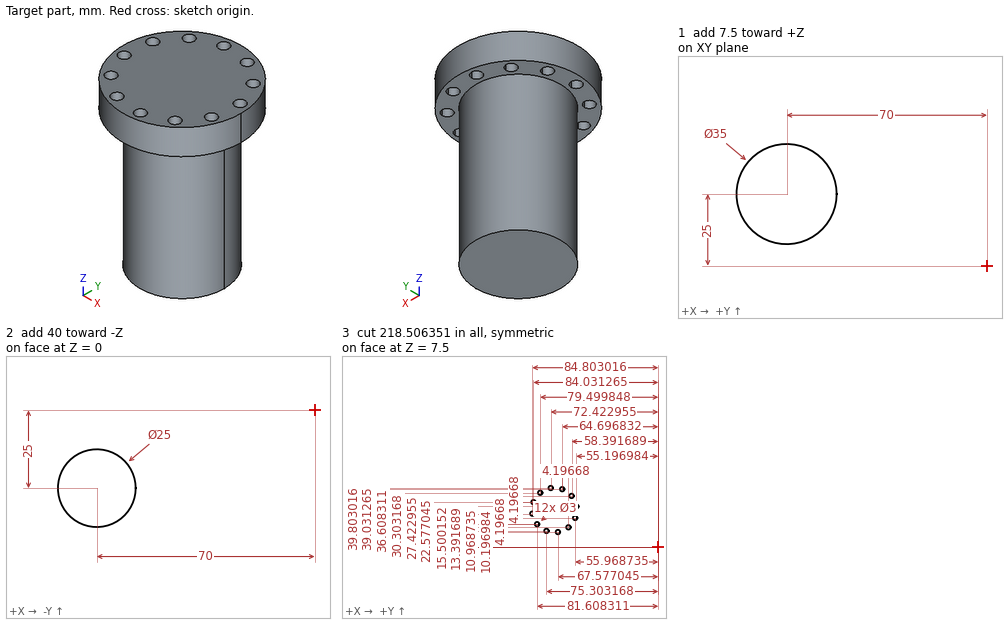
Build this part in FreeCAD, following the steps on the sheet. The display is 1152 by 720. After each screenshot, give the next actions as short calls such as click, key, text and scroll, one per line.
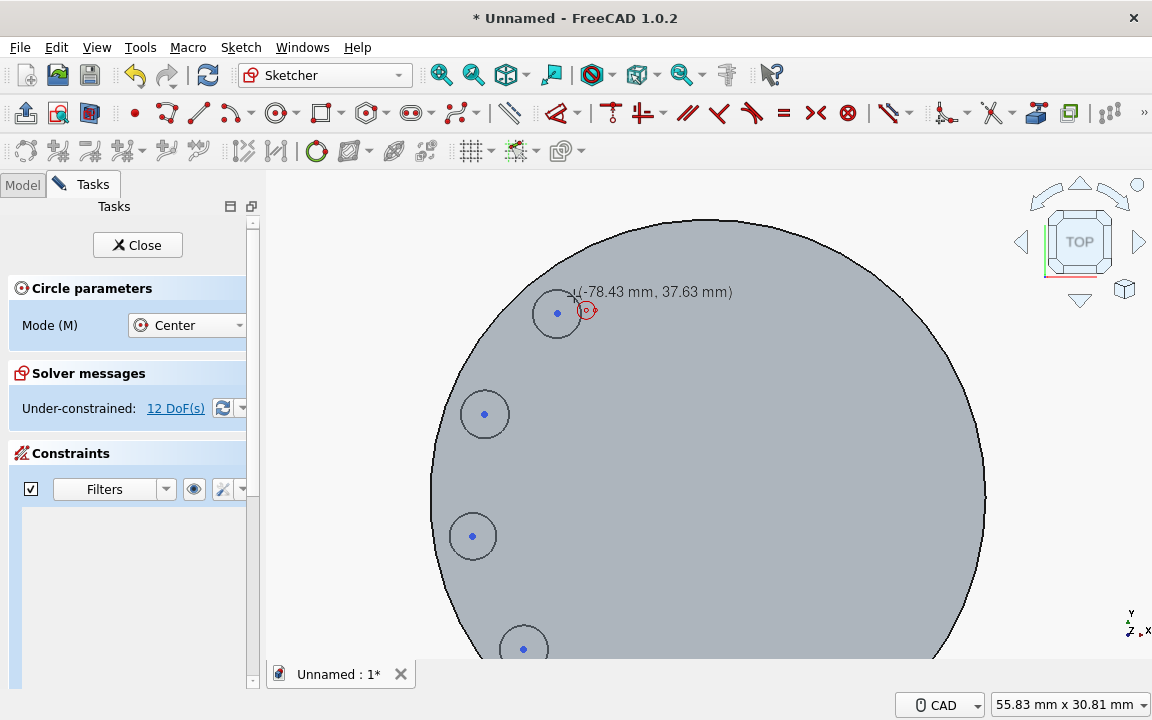
click(669, 262)
click(686, 246)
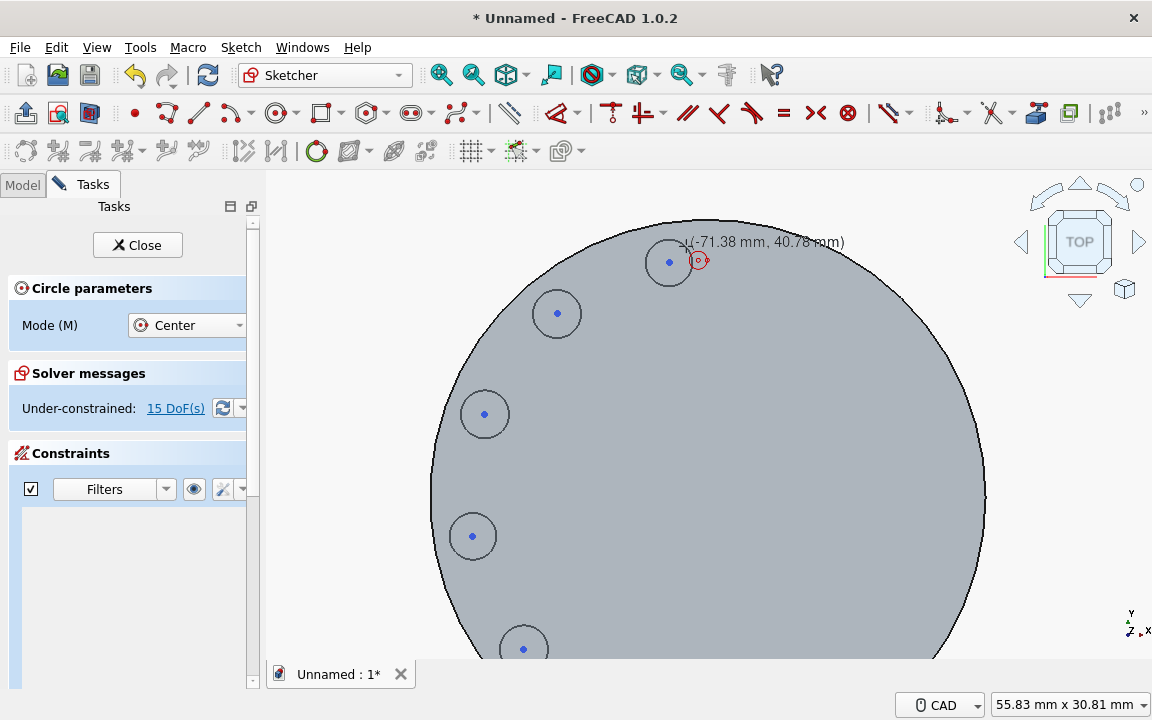
click(792, 275)
click(809, 258)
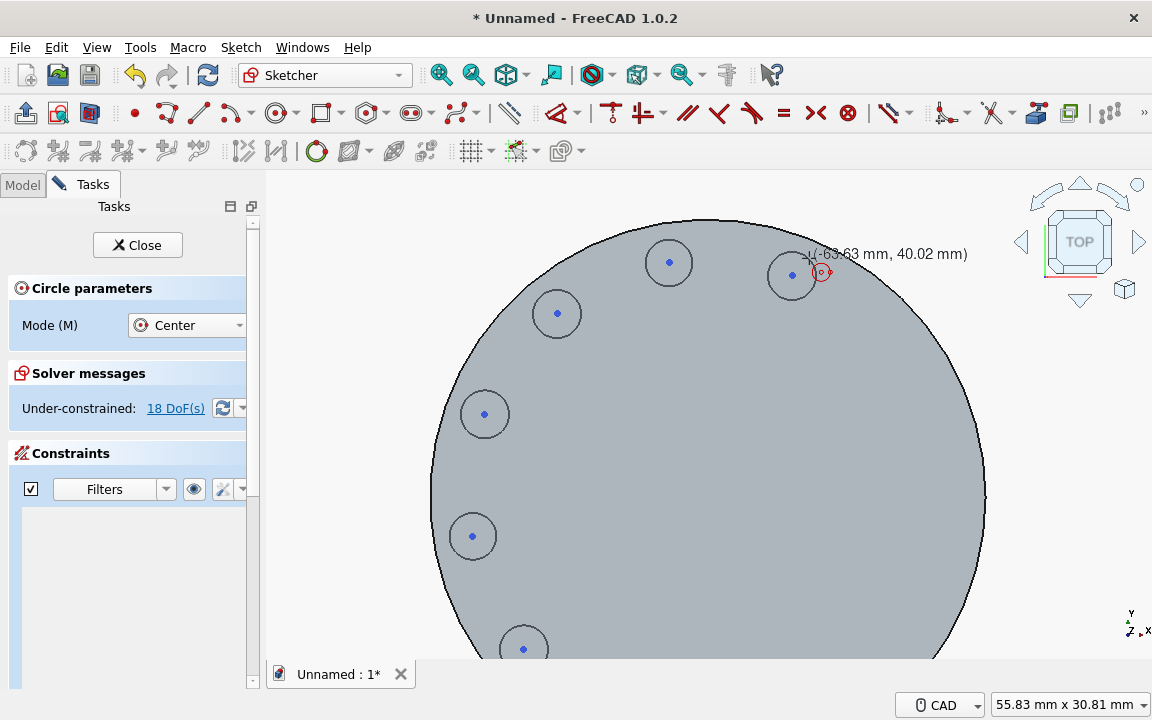
click(892, 347)
click(909, 330)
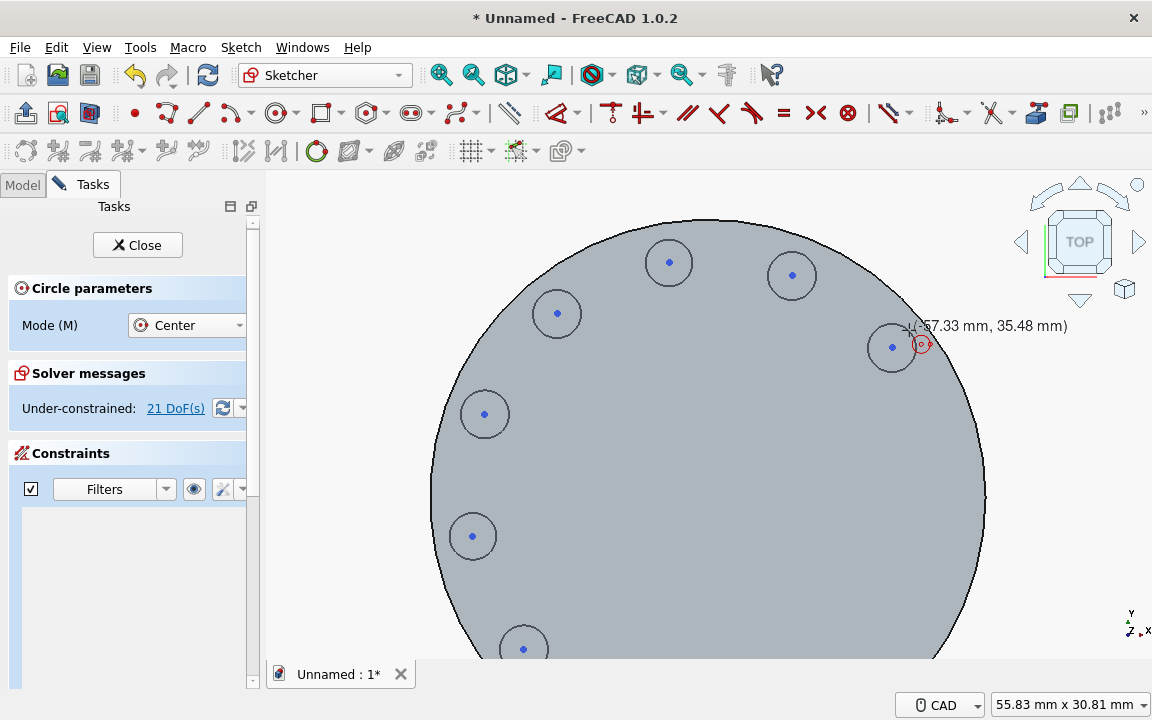
click(943, 459)
click(960, 442)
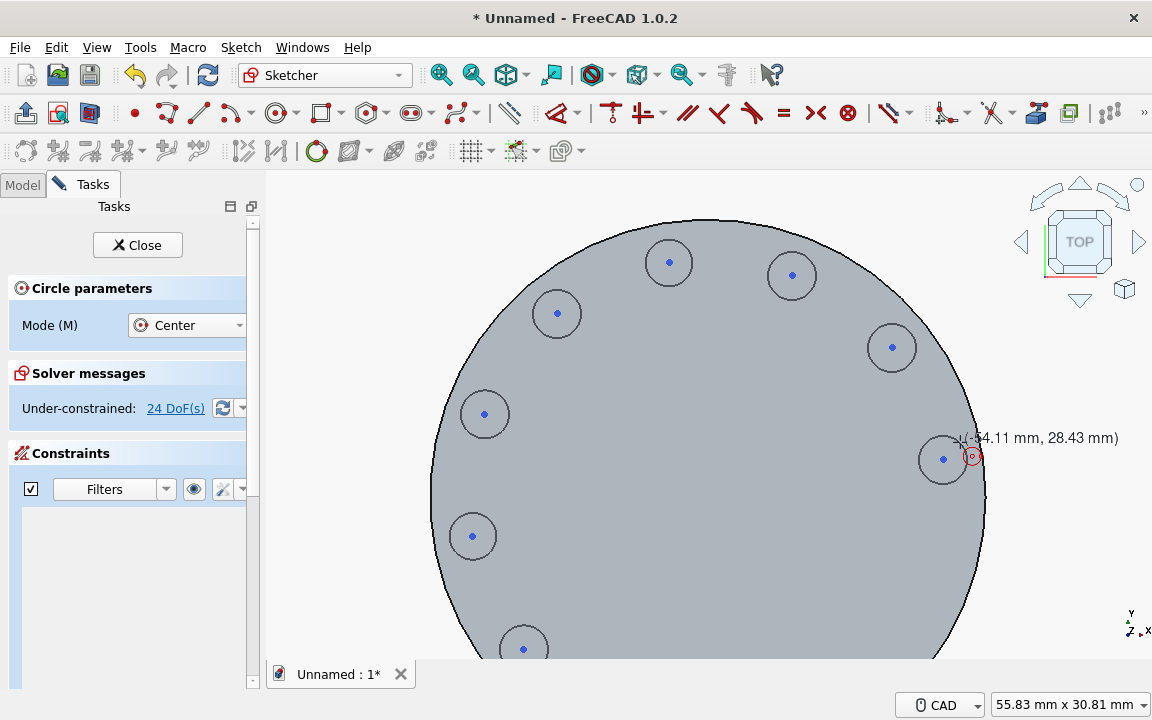
click(931, 582)
click(947, 565)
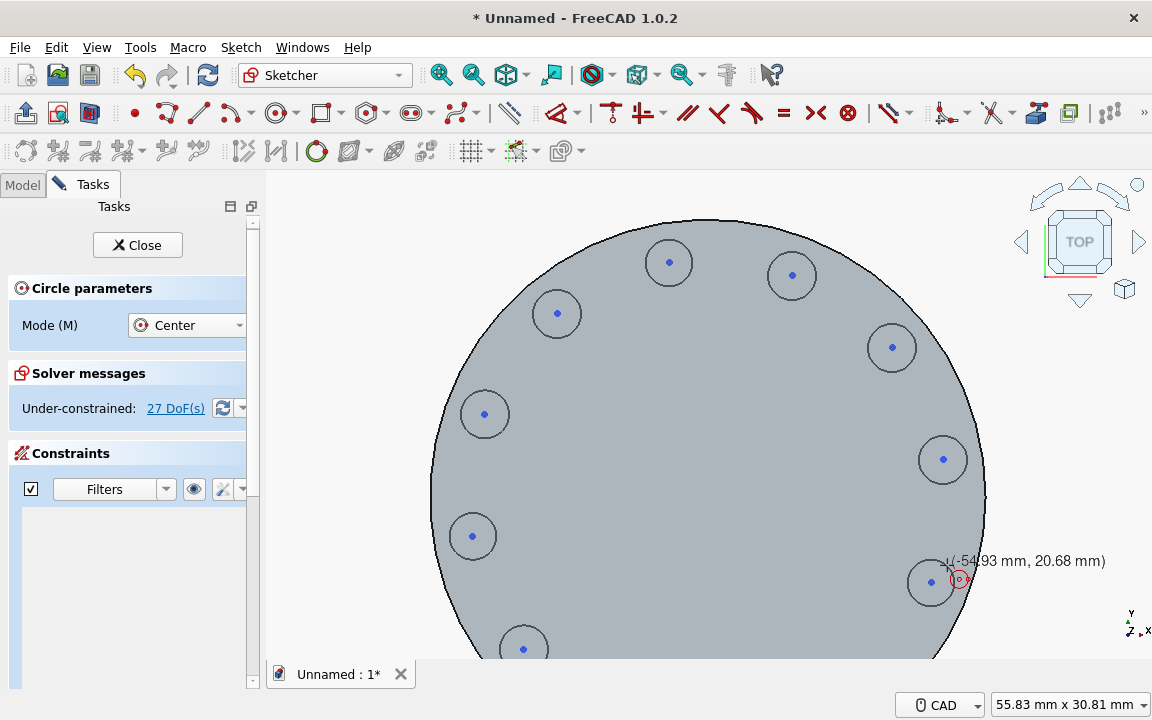
scroll(559, 314, down, 3)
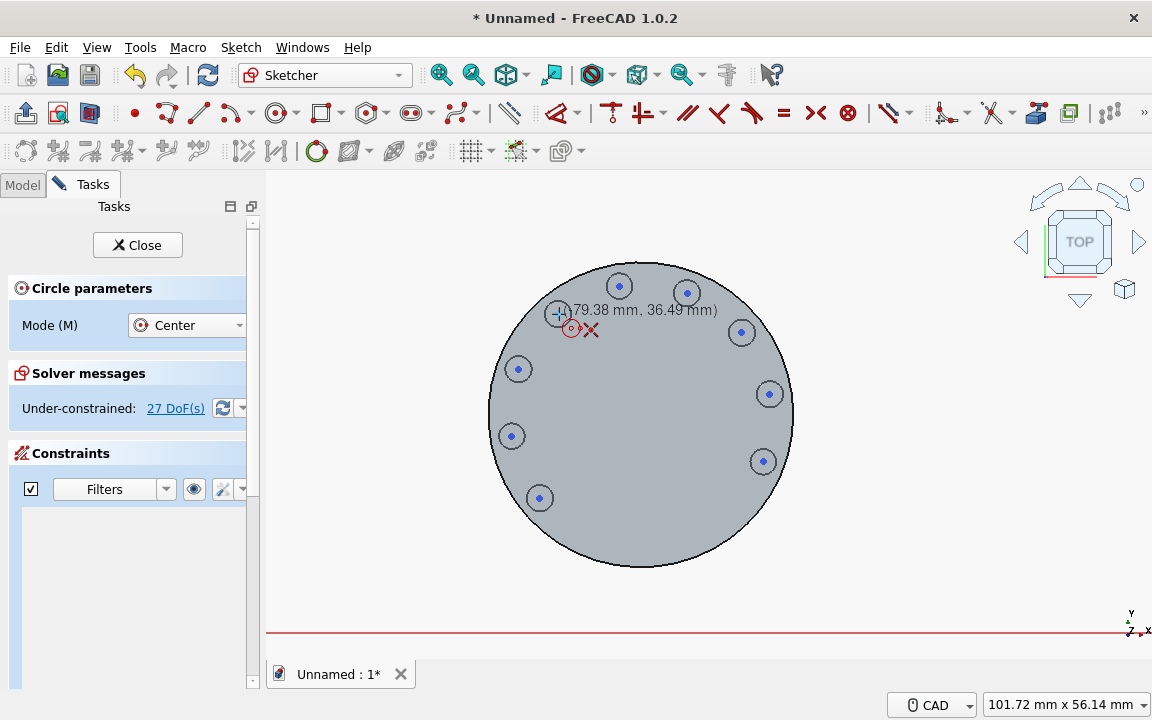
scroll(724, 516, up, 3)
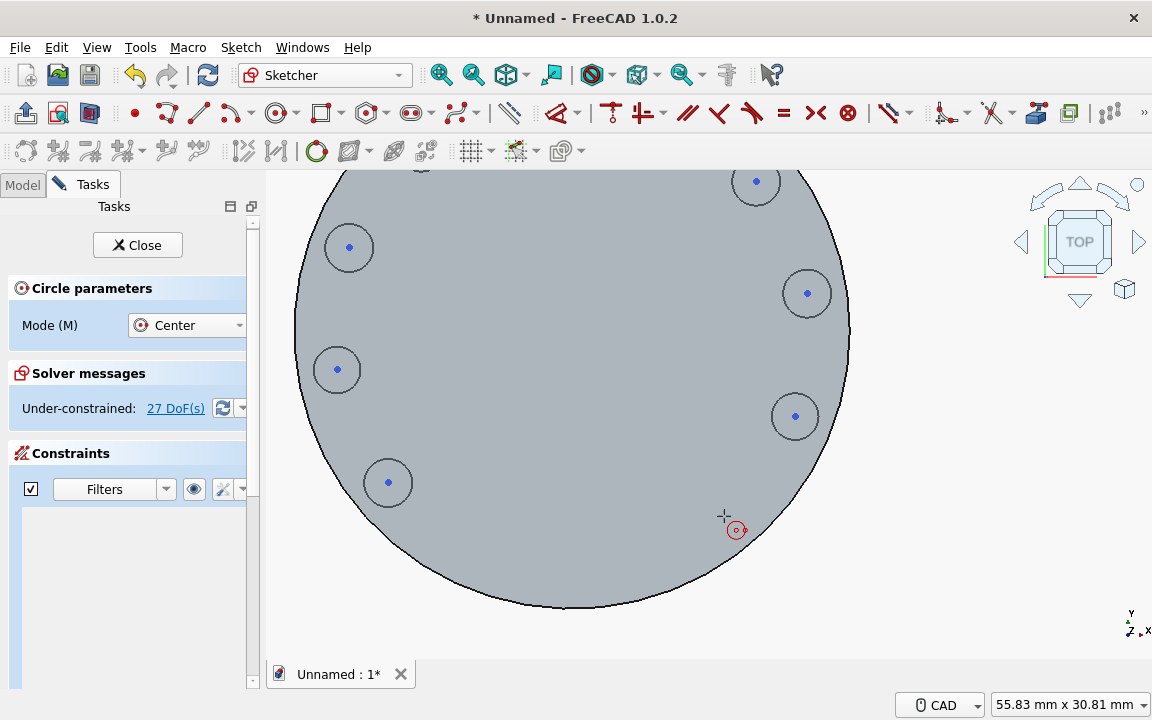
click(723, 515)
click(740, 498)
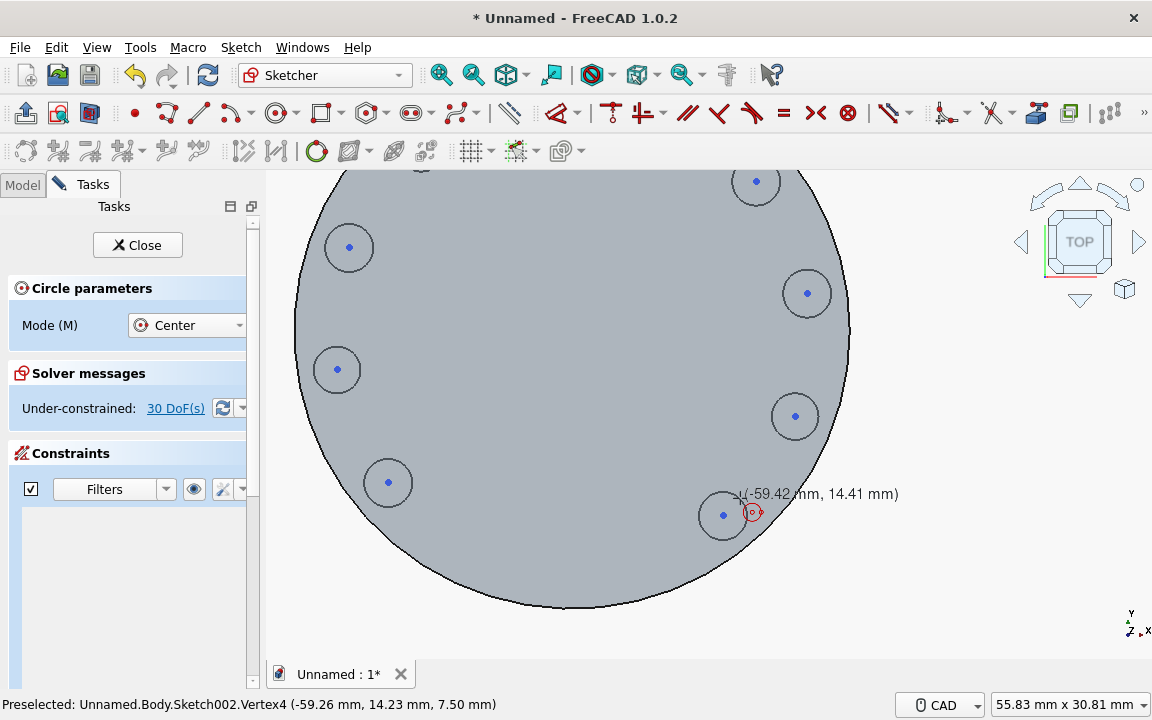
click(611, 566)
click(627, 549)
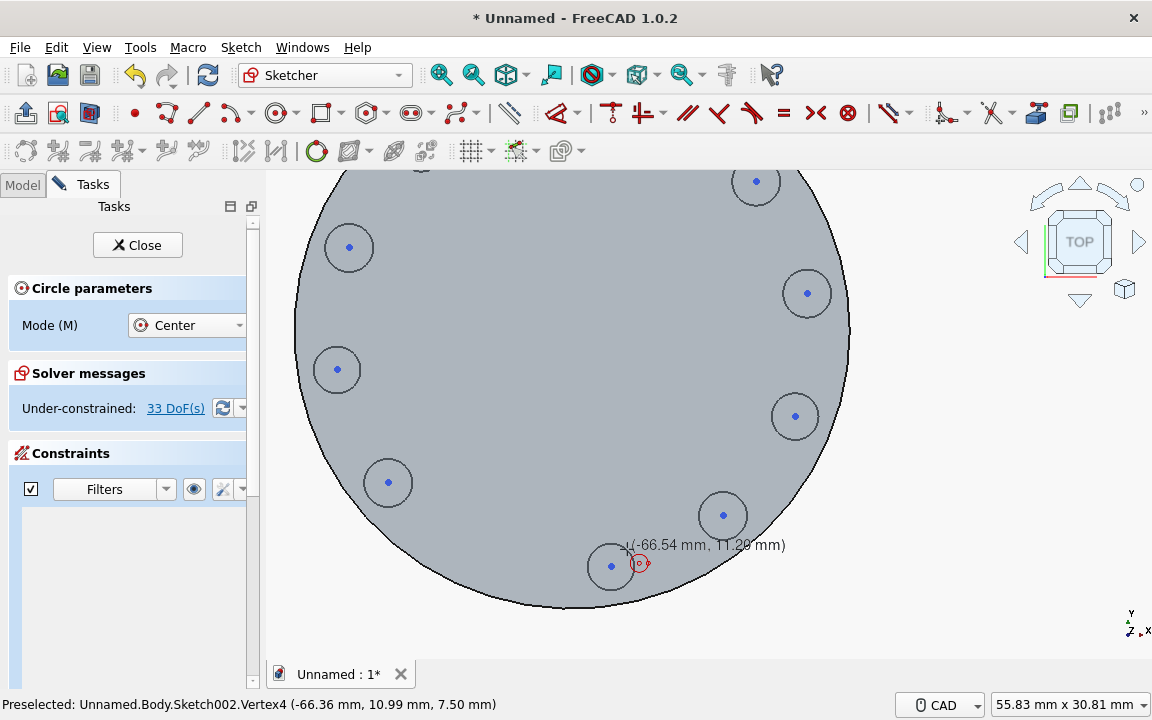
click(488, 554)
click(505, 537)
key(Escape)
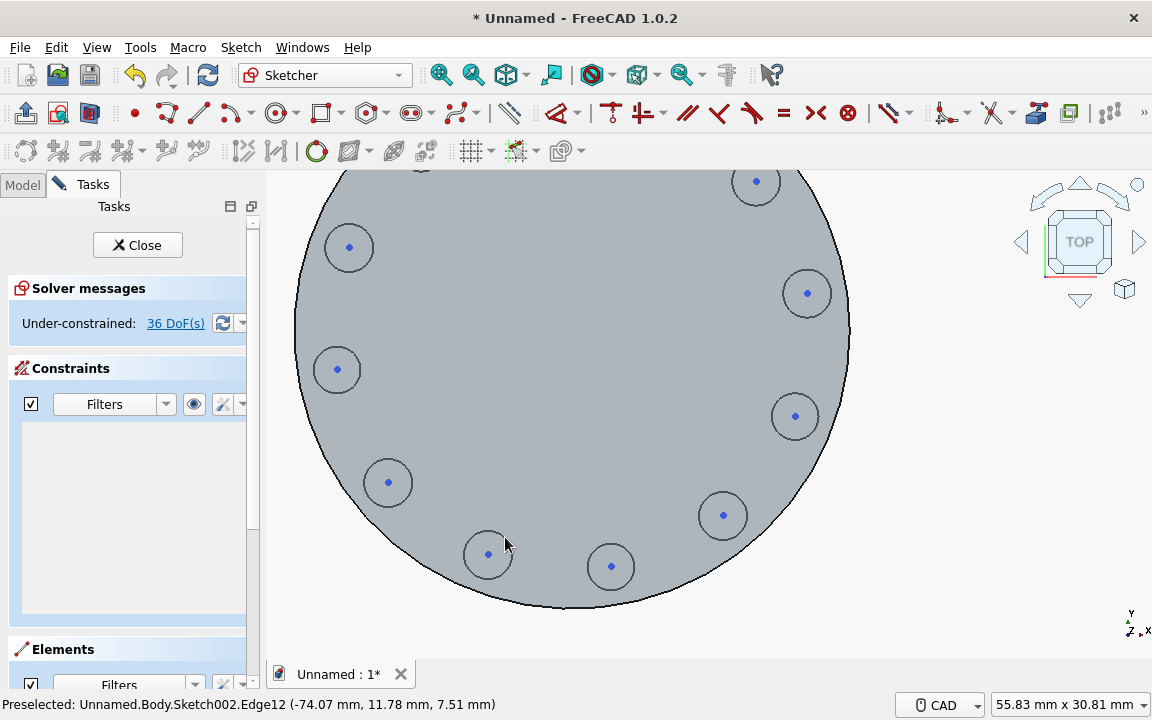
click(405, 466)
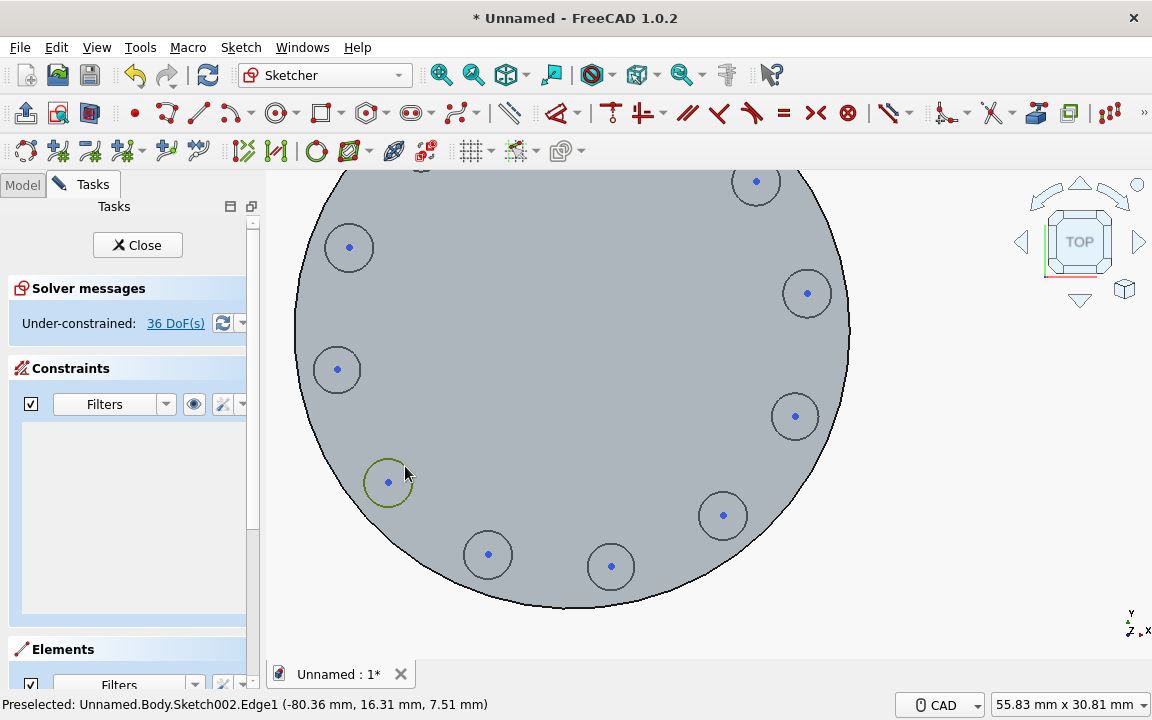
click(354, 353)